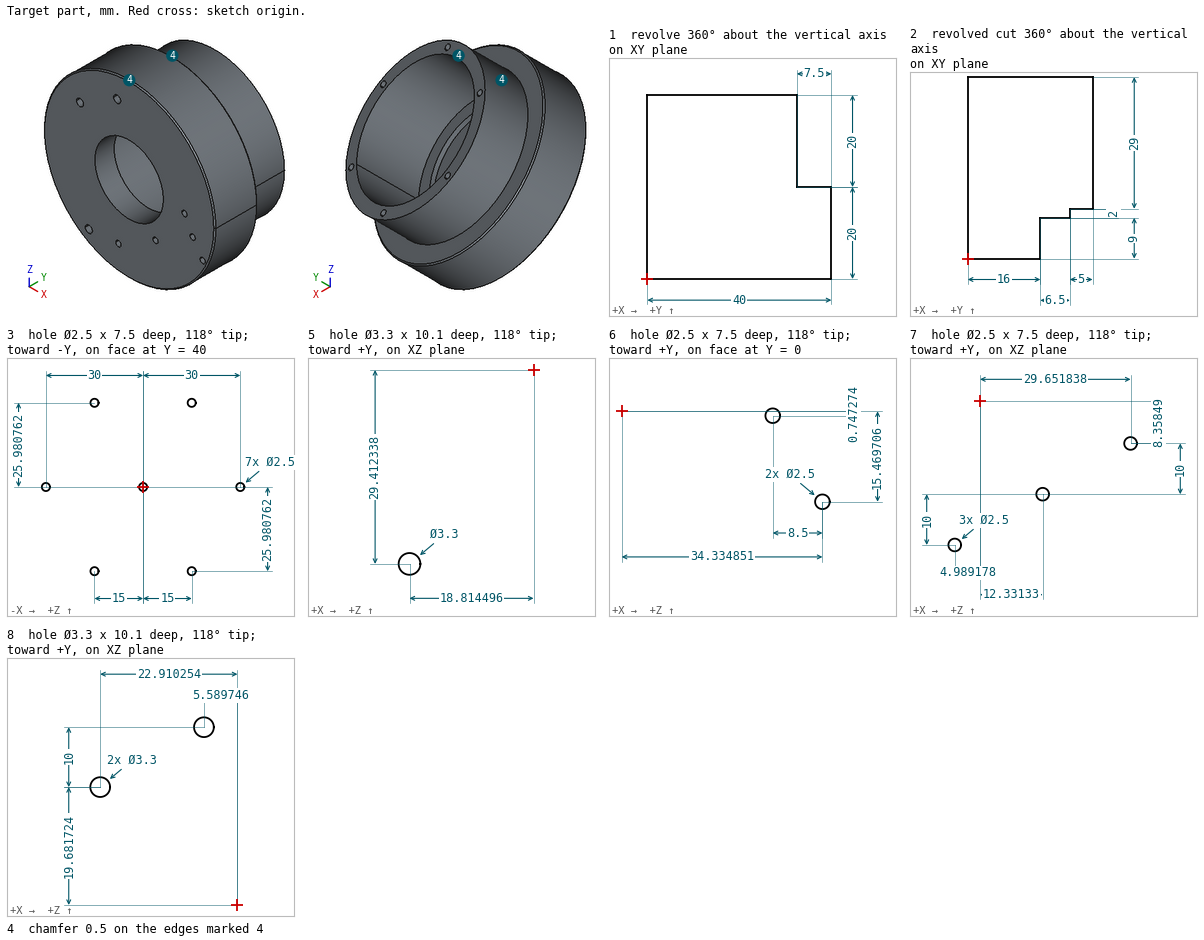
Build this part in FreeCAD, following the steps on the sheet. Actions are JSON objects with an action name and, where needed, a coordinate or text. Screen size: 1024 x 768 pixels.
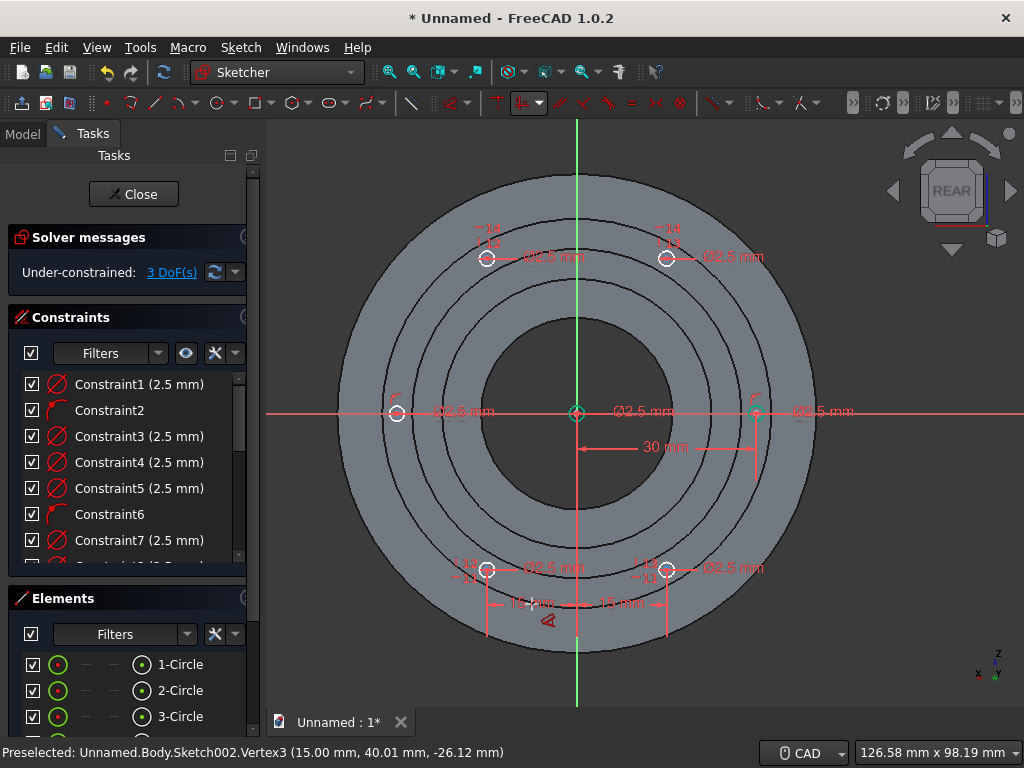
{"action": "left_click", "coordinate": [397, 414]}
{"action": "left_click", "coordinate": [487, 448]}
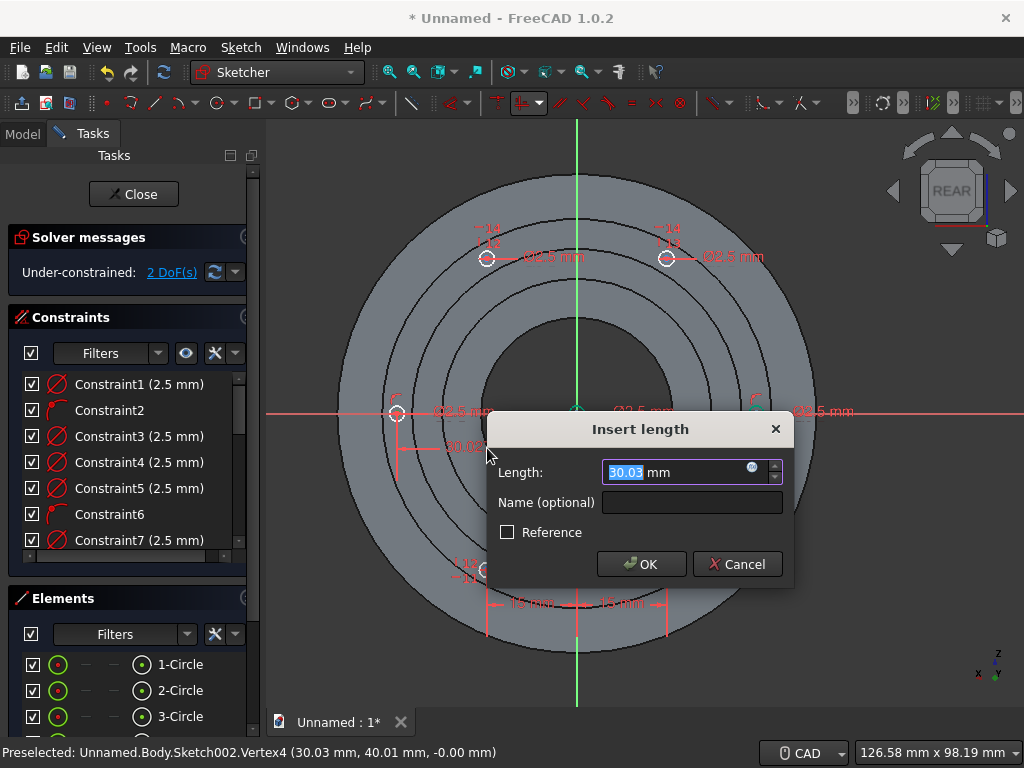
{"action": "type", "text": "30"}
{"action": "key", "text": "Return"}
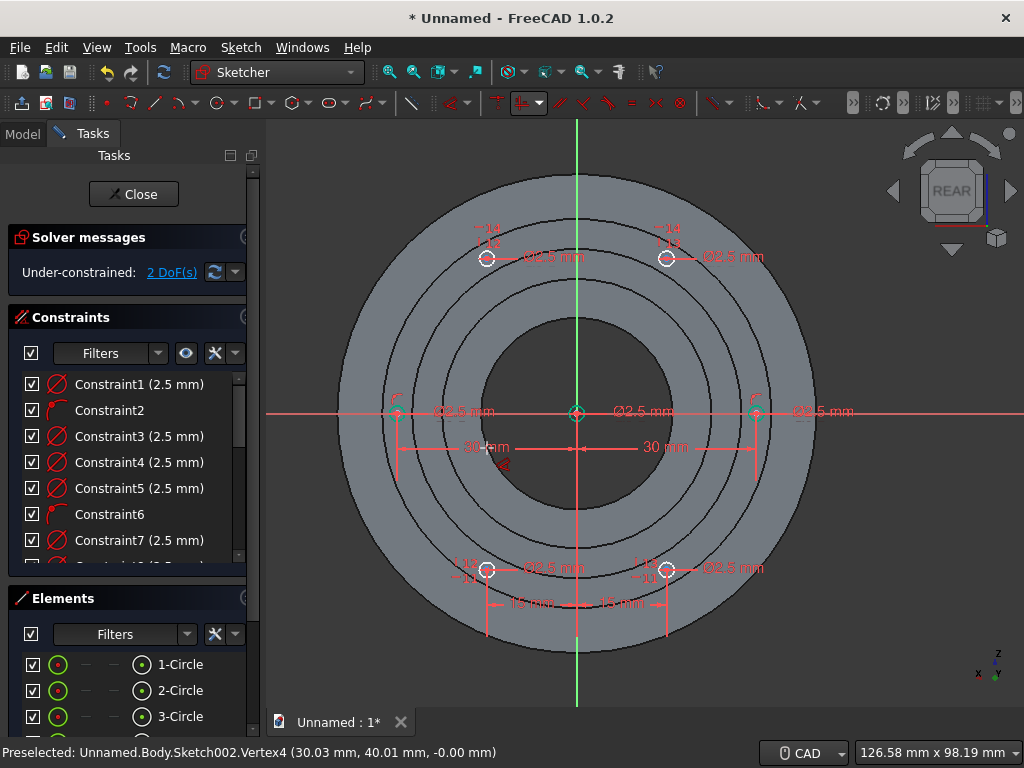
{"action": "left_click", "coordinate": [667, 570]}
{"action": "left_click", "coordinate": [701, 492]}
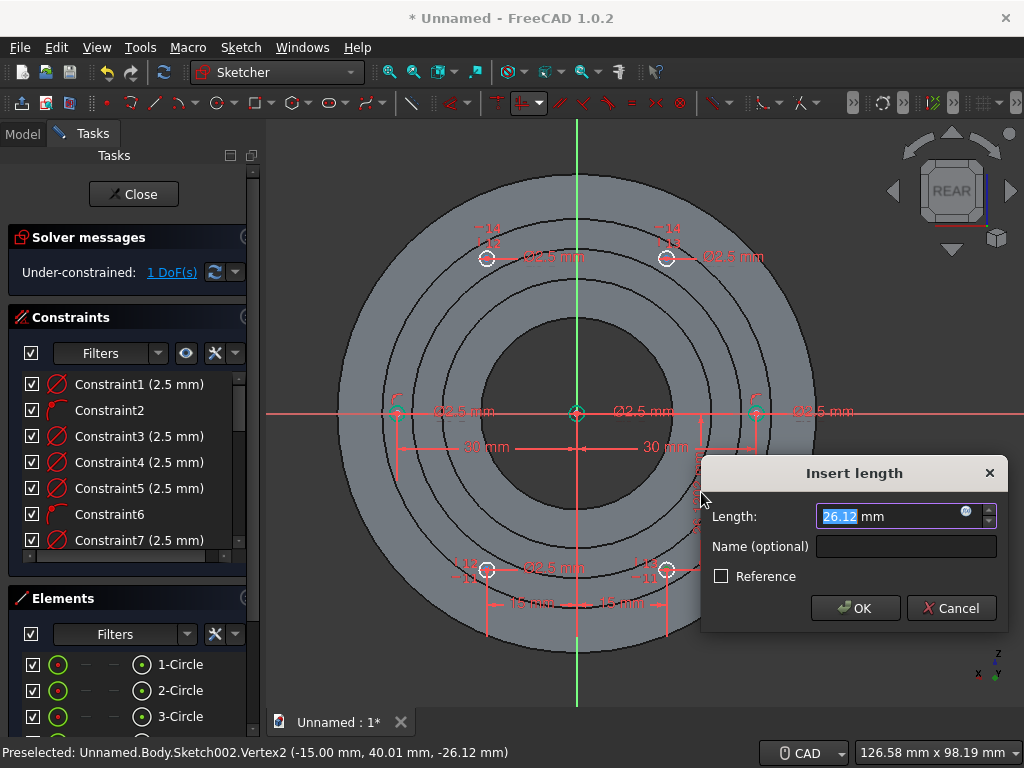
{"action": "type", "text": "25.980762"}
{"action": "key", "text": "Return"}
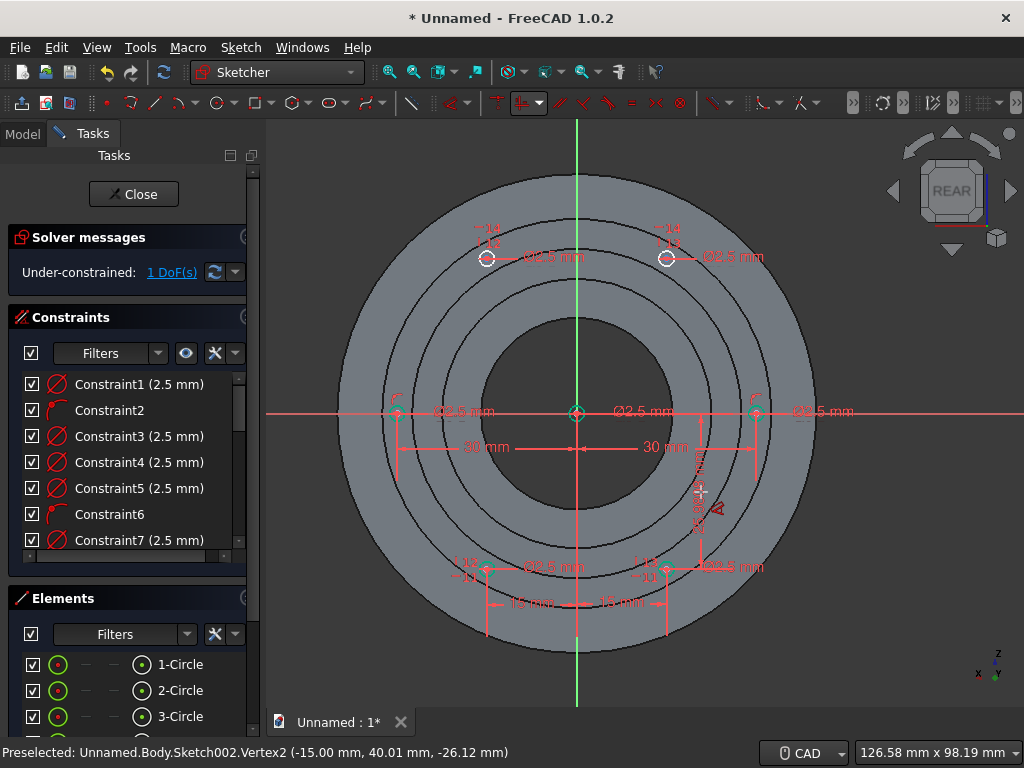
{"action": "left_click", "coordinate": [487, 259]}
{"action": "left_click", "coordinate": [453, 336]}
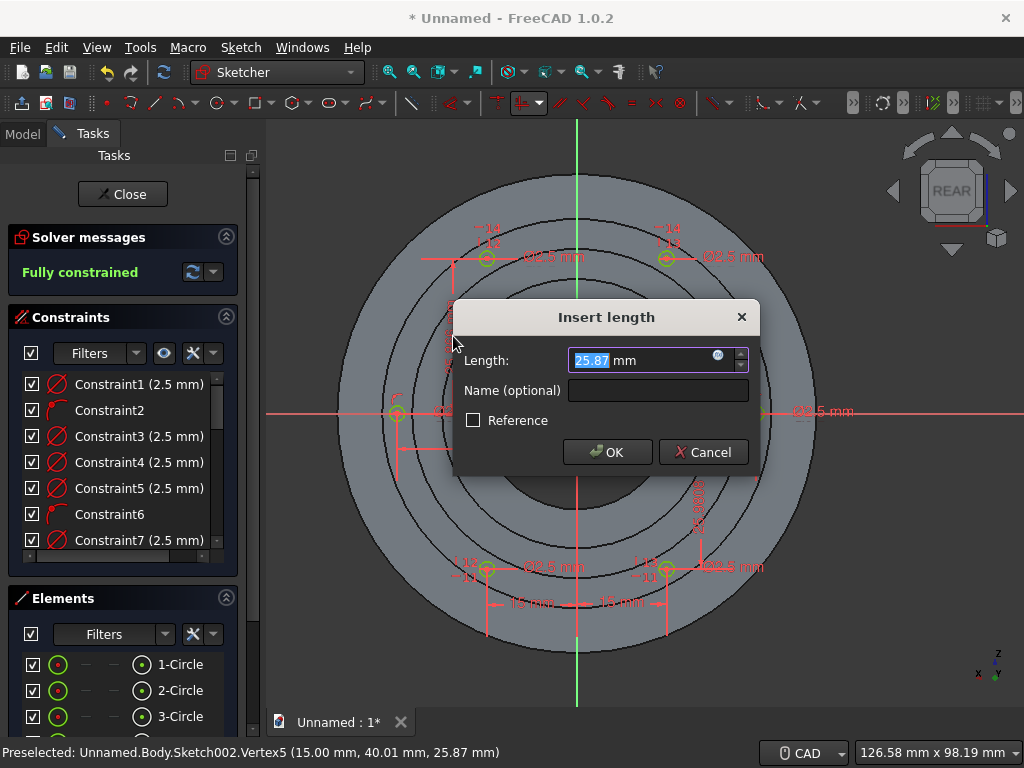
{"action": "type", "text": "25.980762"}
{"action": "key", "text": "Return"}
{"action": "key", "text": "Escape"}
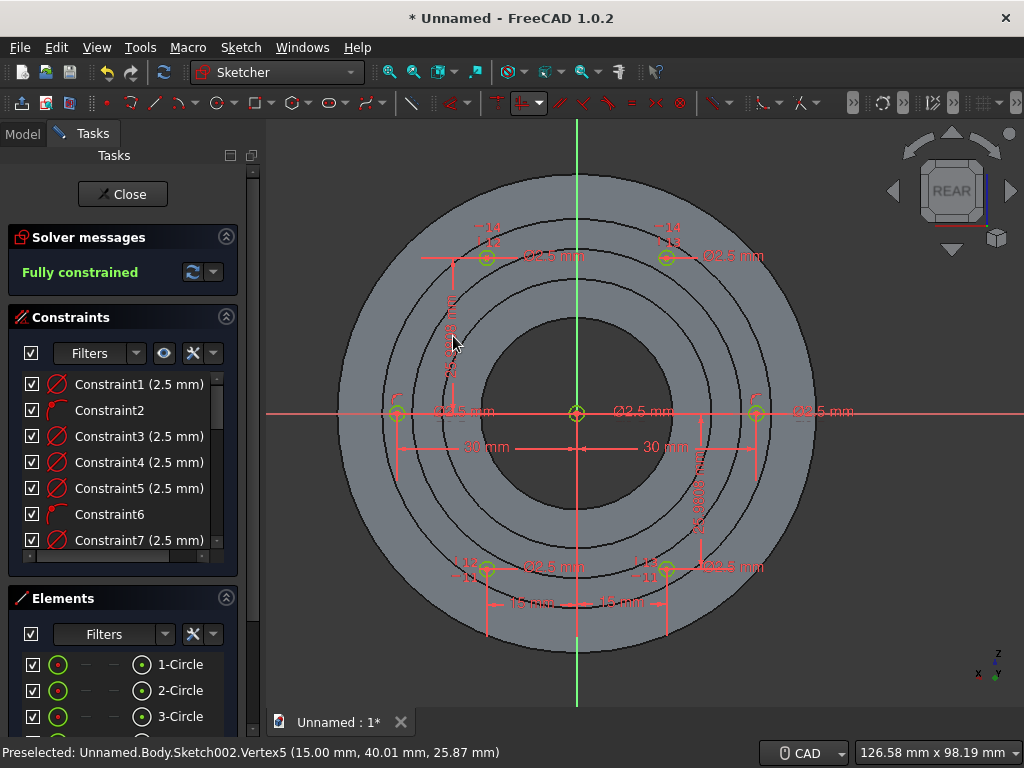
{"action": "left_click", "coordinate": [123, 194]}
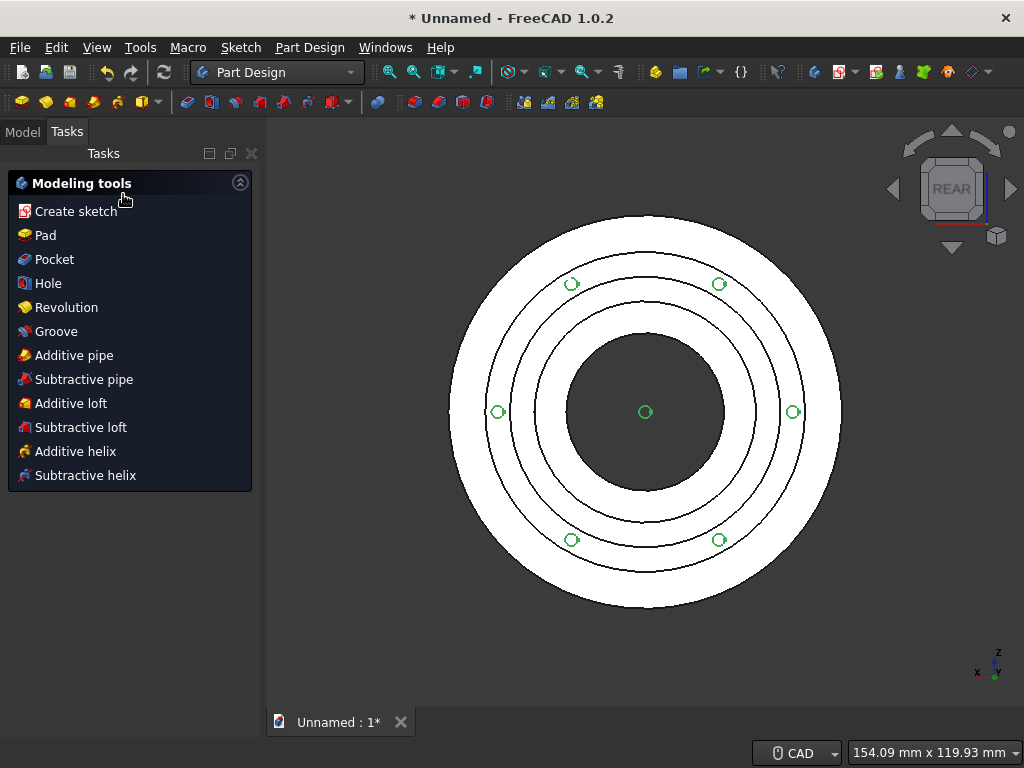
{"action": "left_click", "coordinate": [212, 102]}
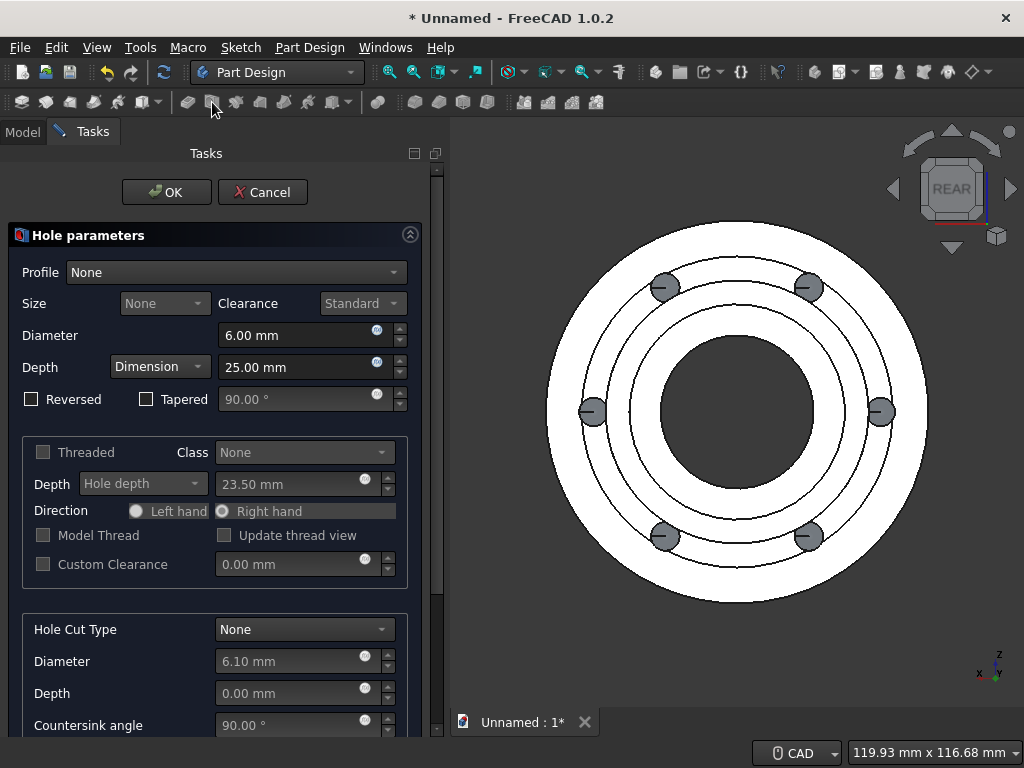
{"action": "triple_click", "coordinate": [305, 335]}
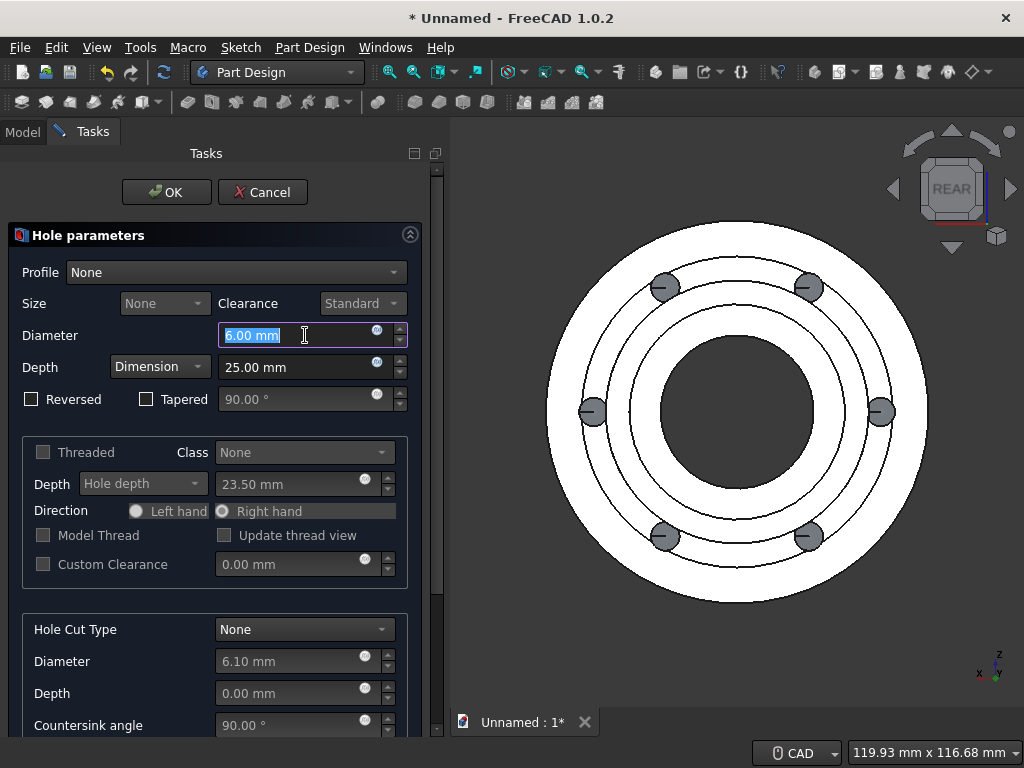
{"action": "type", "text": "2.5"}
{"action": "key", "text": "Tab"}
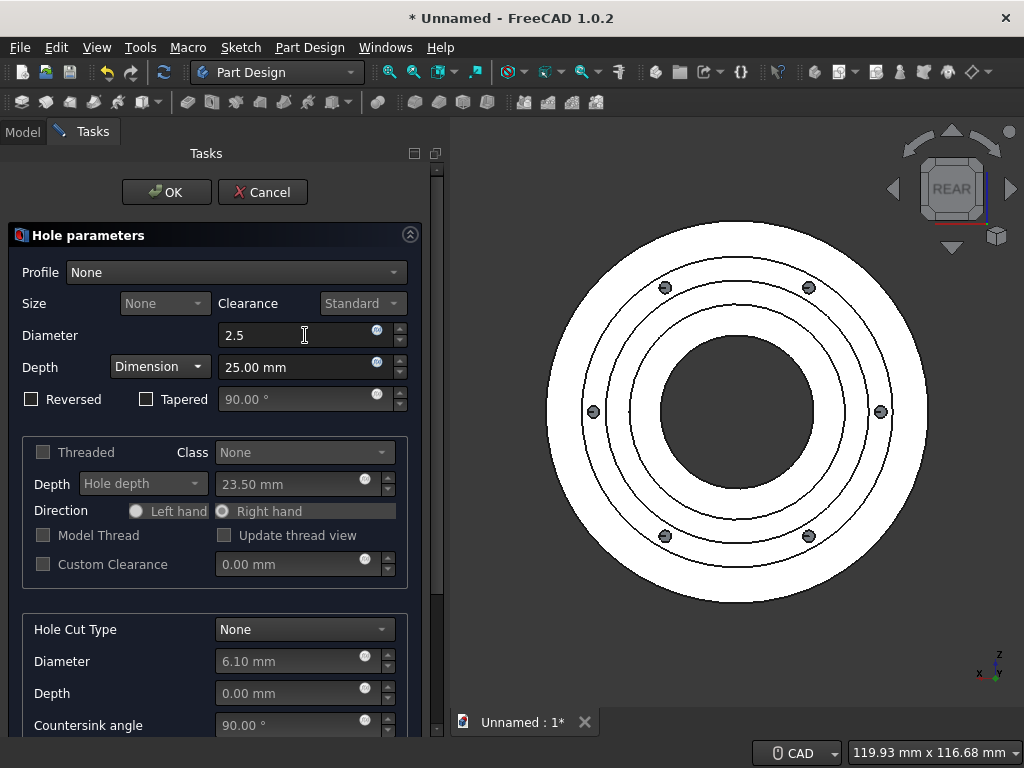
{"action": "triple_click", "coordinate": [305, 367]}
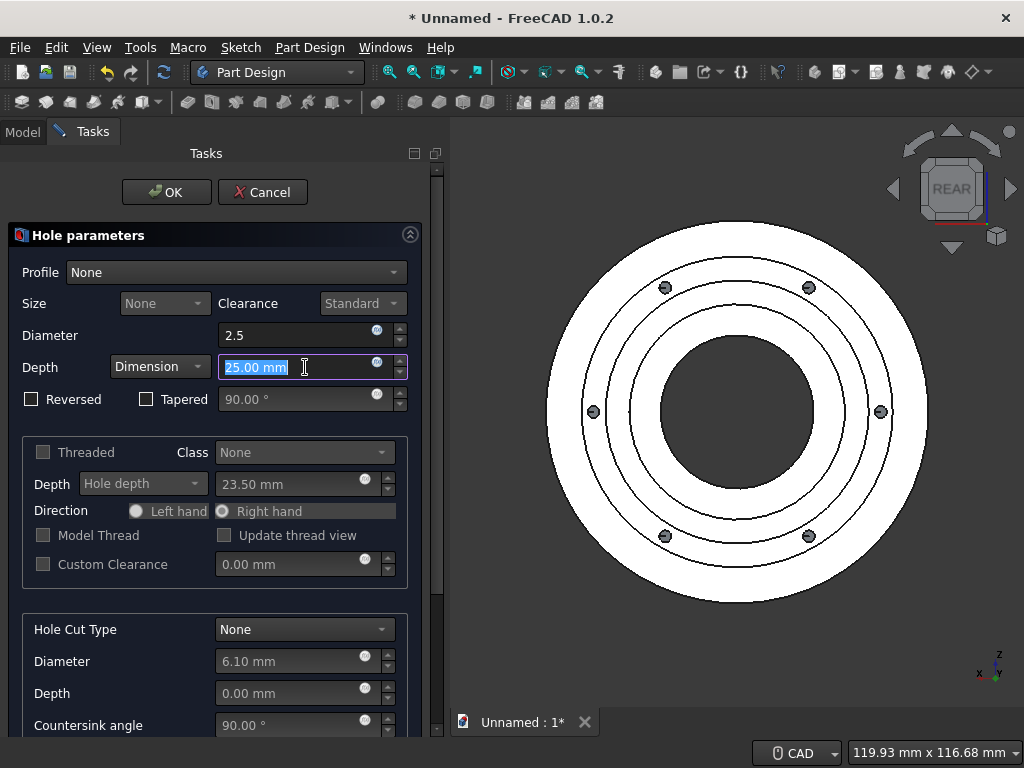
{"action": "type", "text": "7.5"}
{"action": "key", "text": "Tab"}